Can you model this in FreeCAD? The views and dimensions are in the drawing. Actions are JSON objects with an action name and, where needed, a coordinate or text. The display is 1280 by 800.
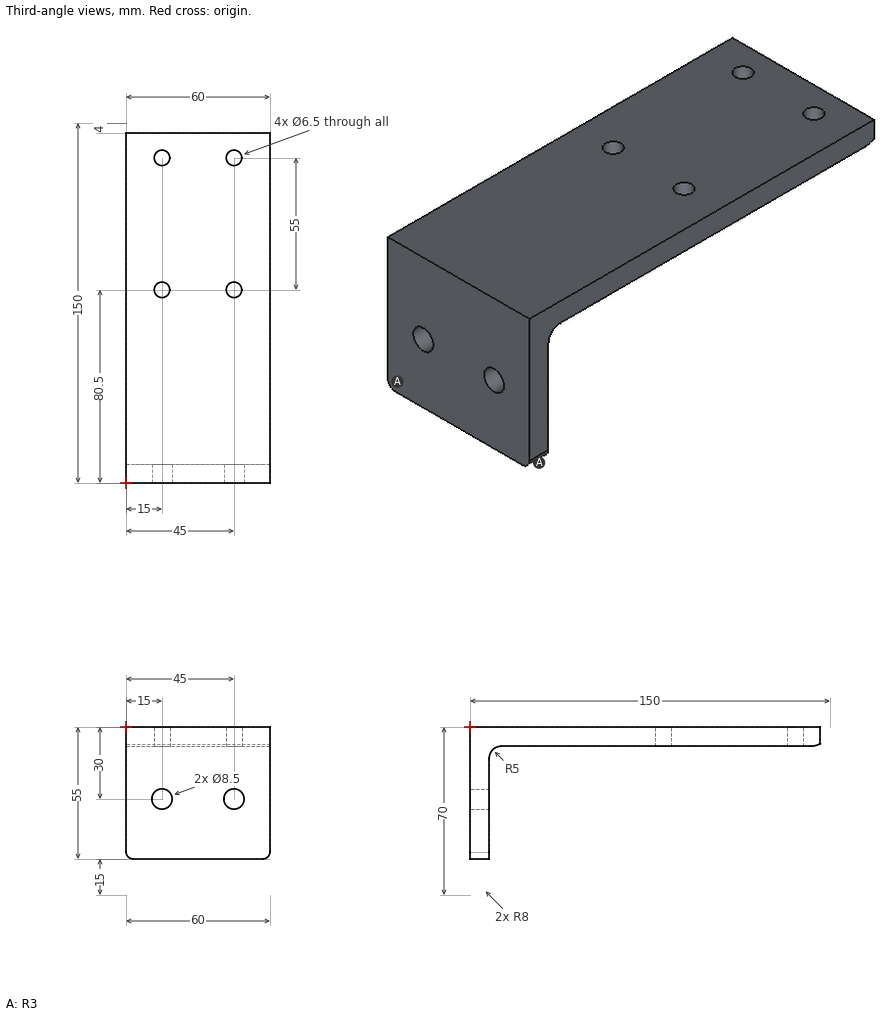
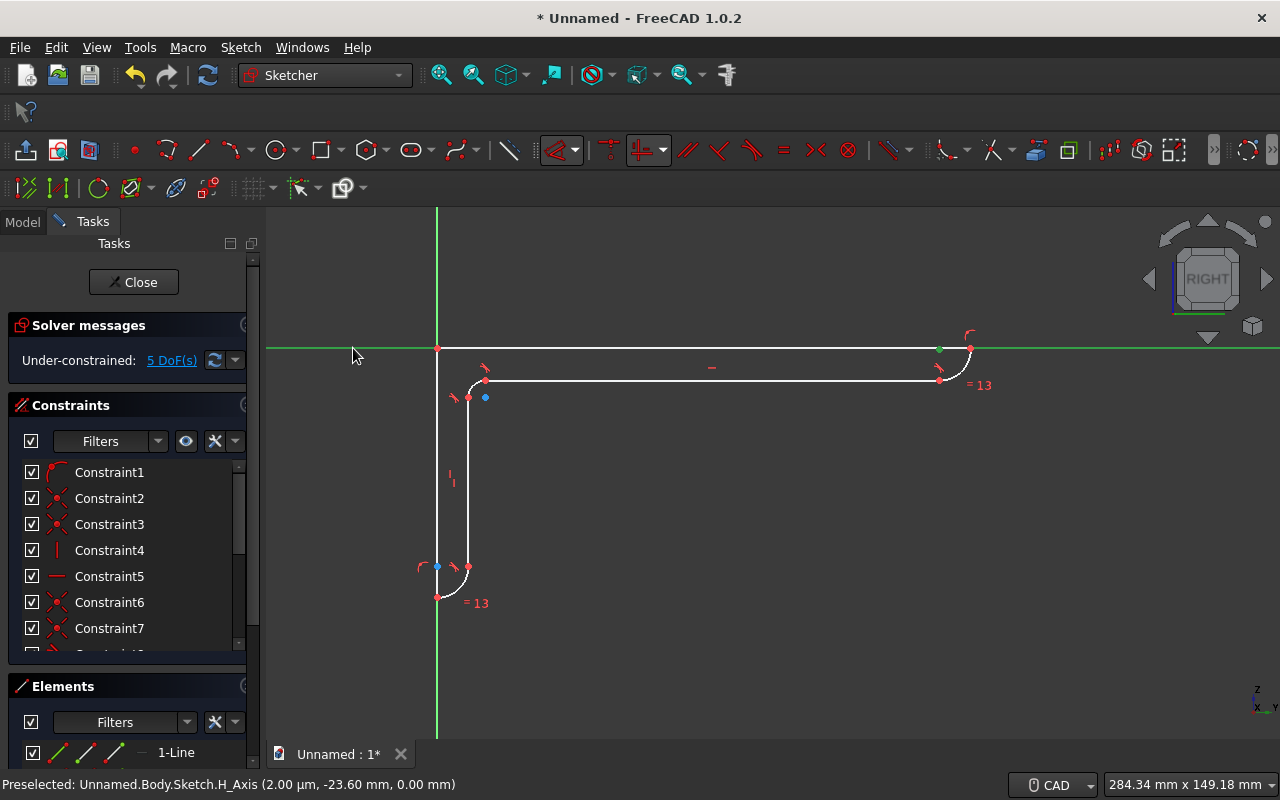
{"action": "key", "text": "c"}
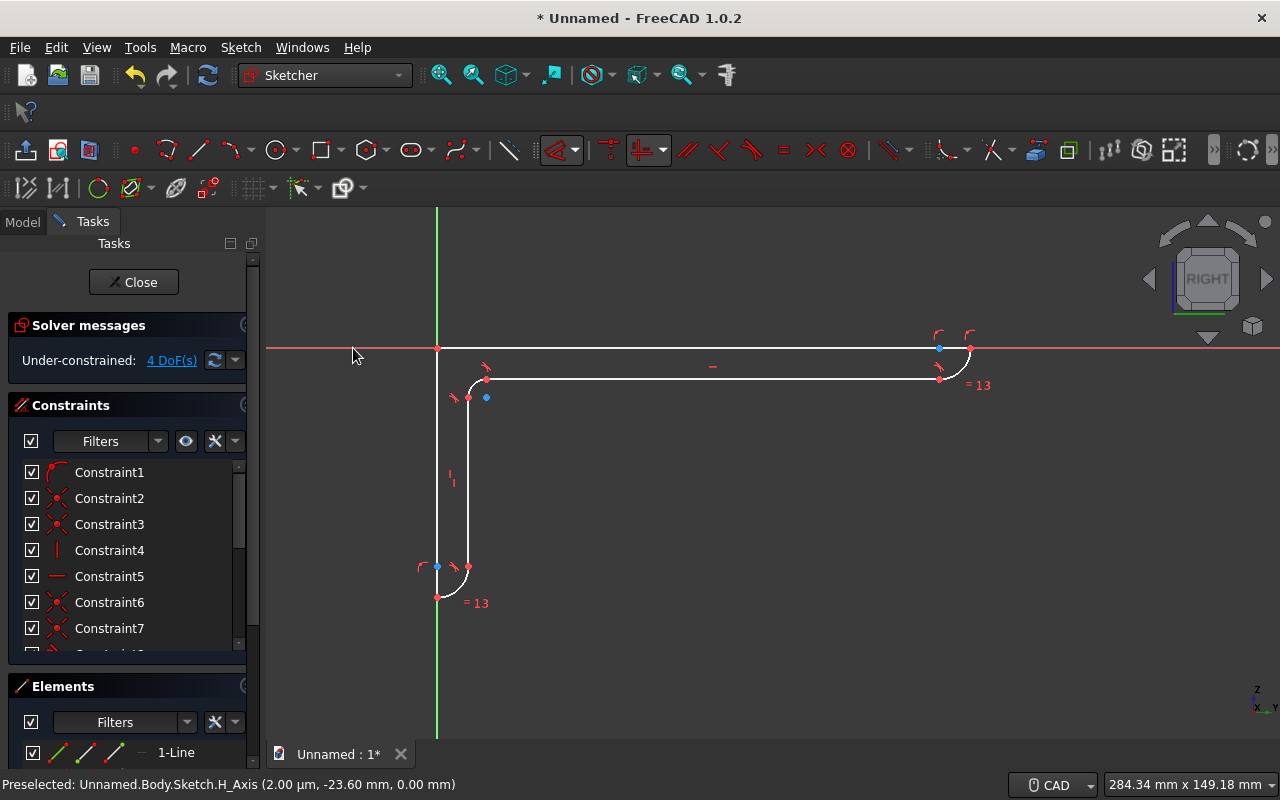
{"action": "key", "text": "d"}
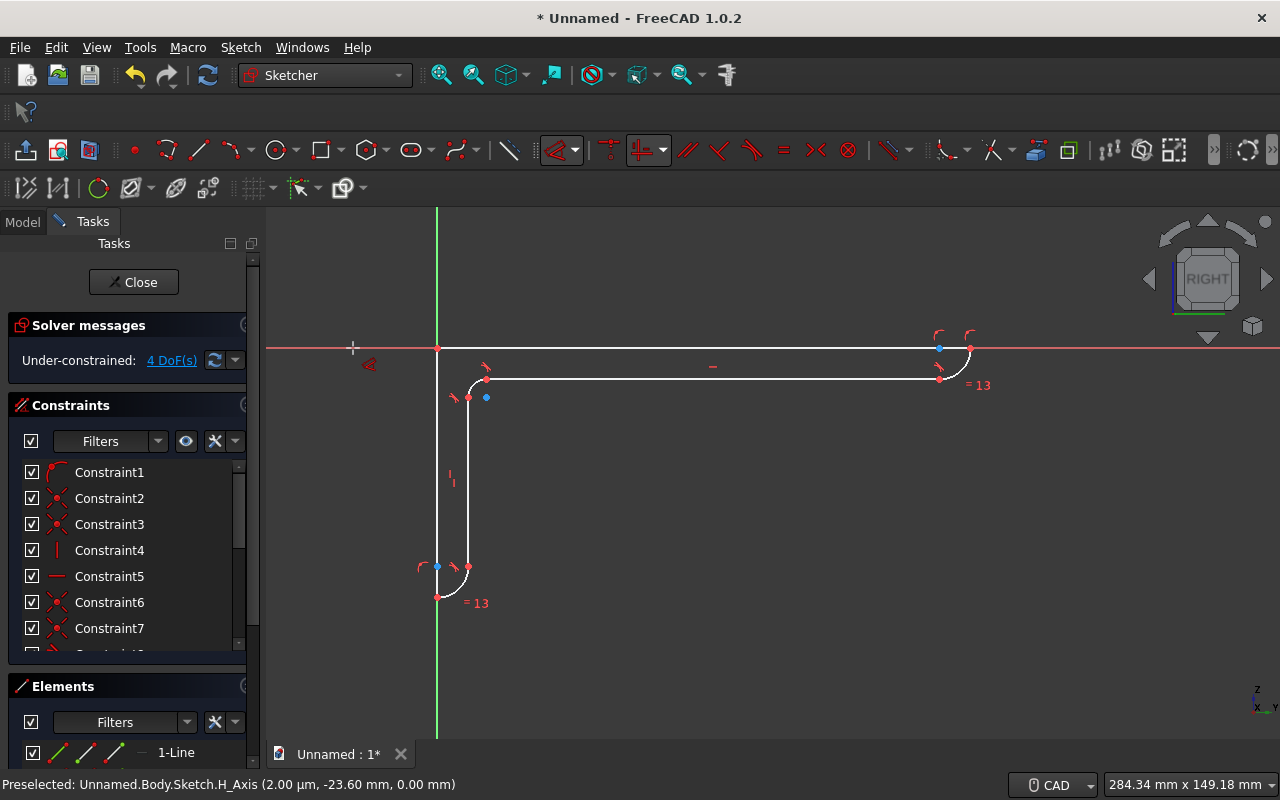
{"action": "scroll", "coordinate": [451, 594], "scroll_direction": "up", "scroll_amount": 2}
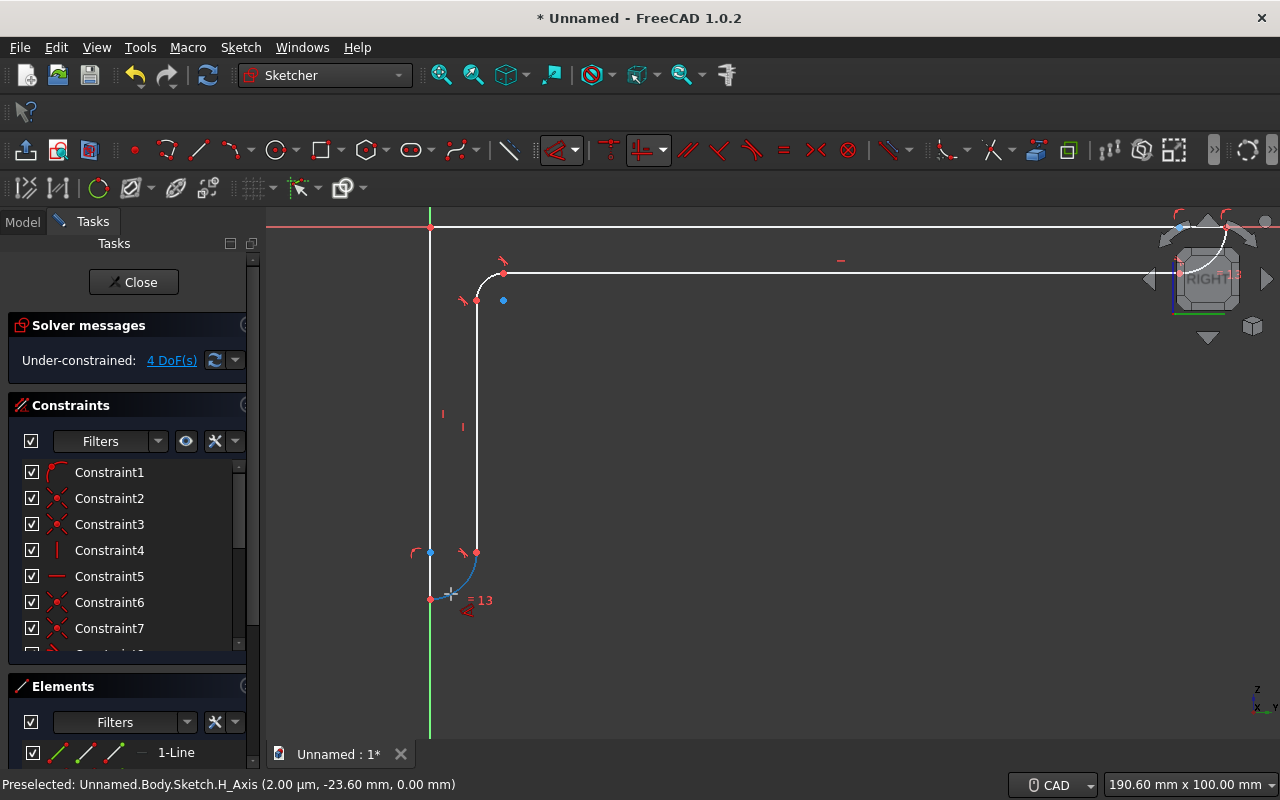
{"action": "left_click", "coordinate": [451, 594]}
{"action": "left_click", "coordinate": [465, 623]}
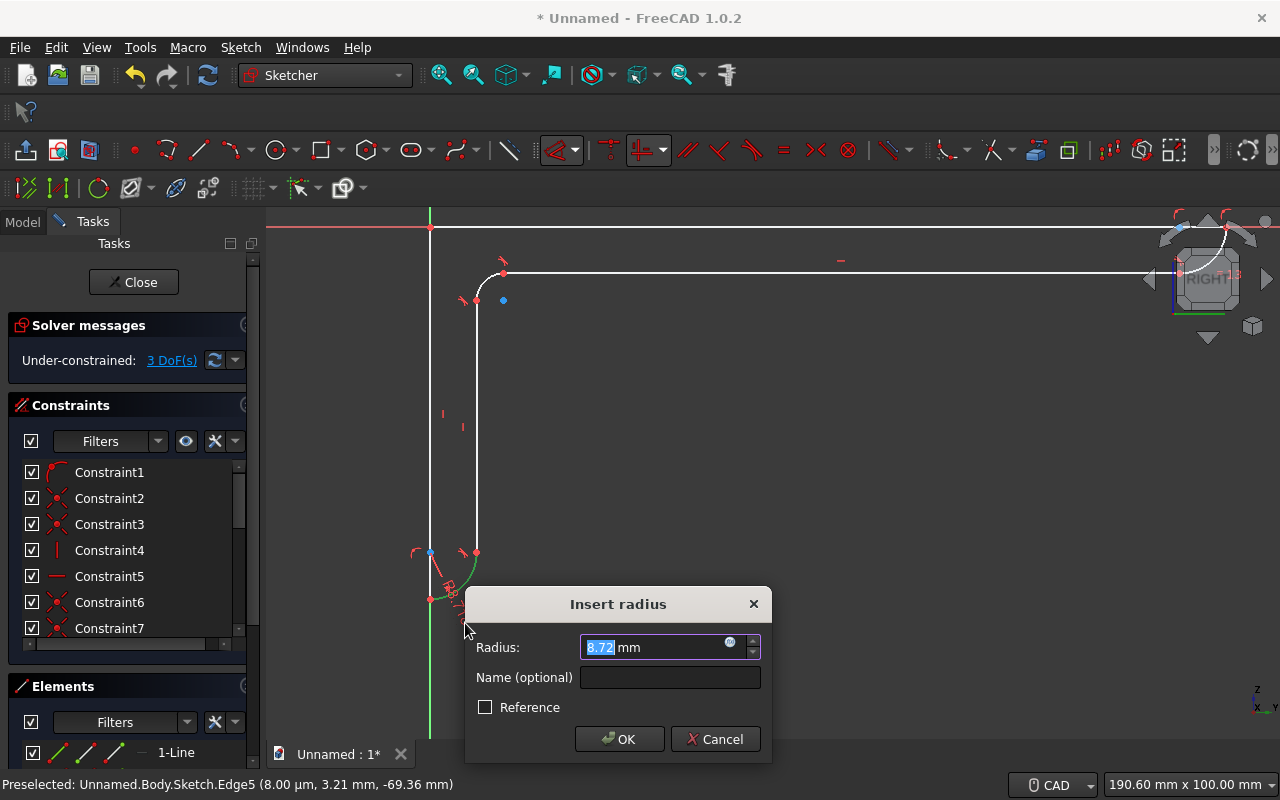
{"action": "type", "text": "8"}
{"action": "key", "text": "Return"}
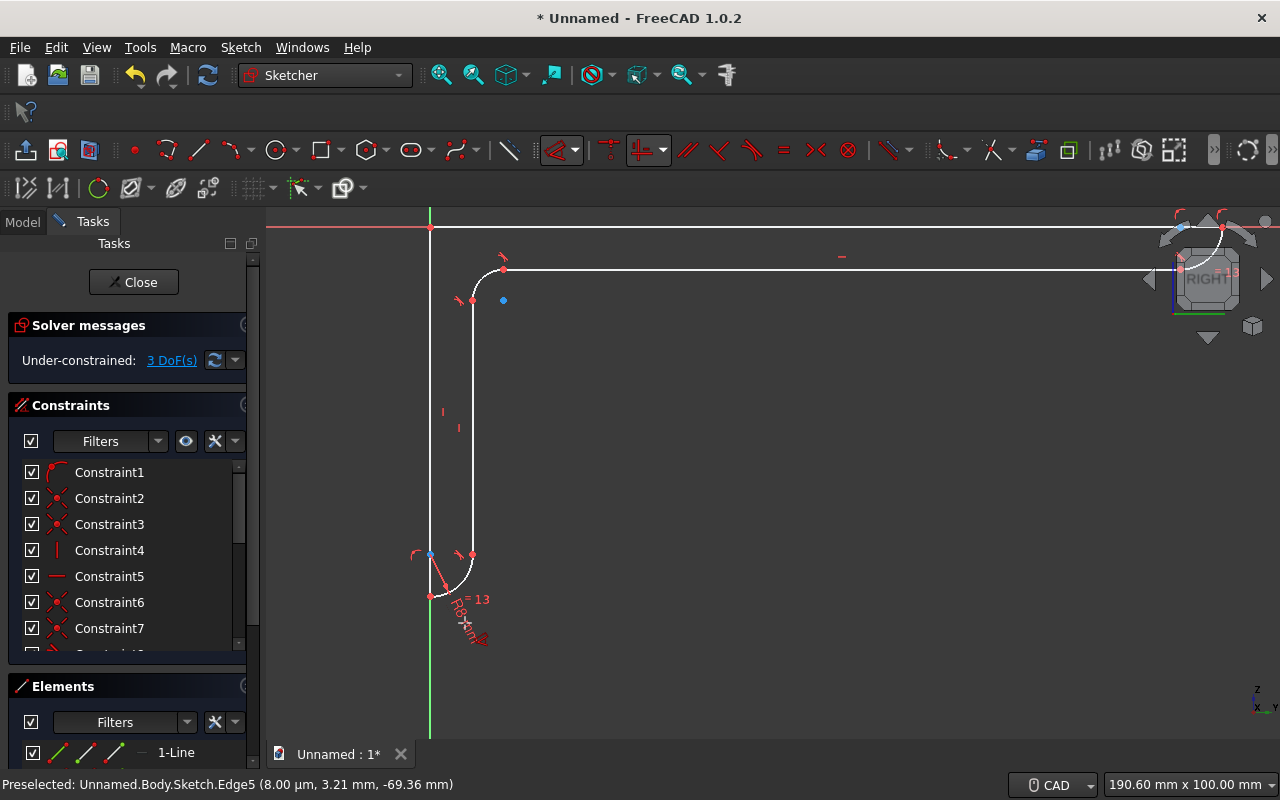
{"action": "scroll", "coordinate": [490, 273], "scroll_direction": "up", "scroll_amount": 3}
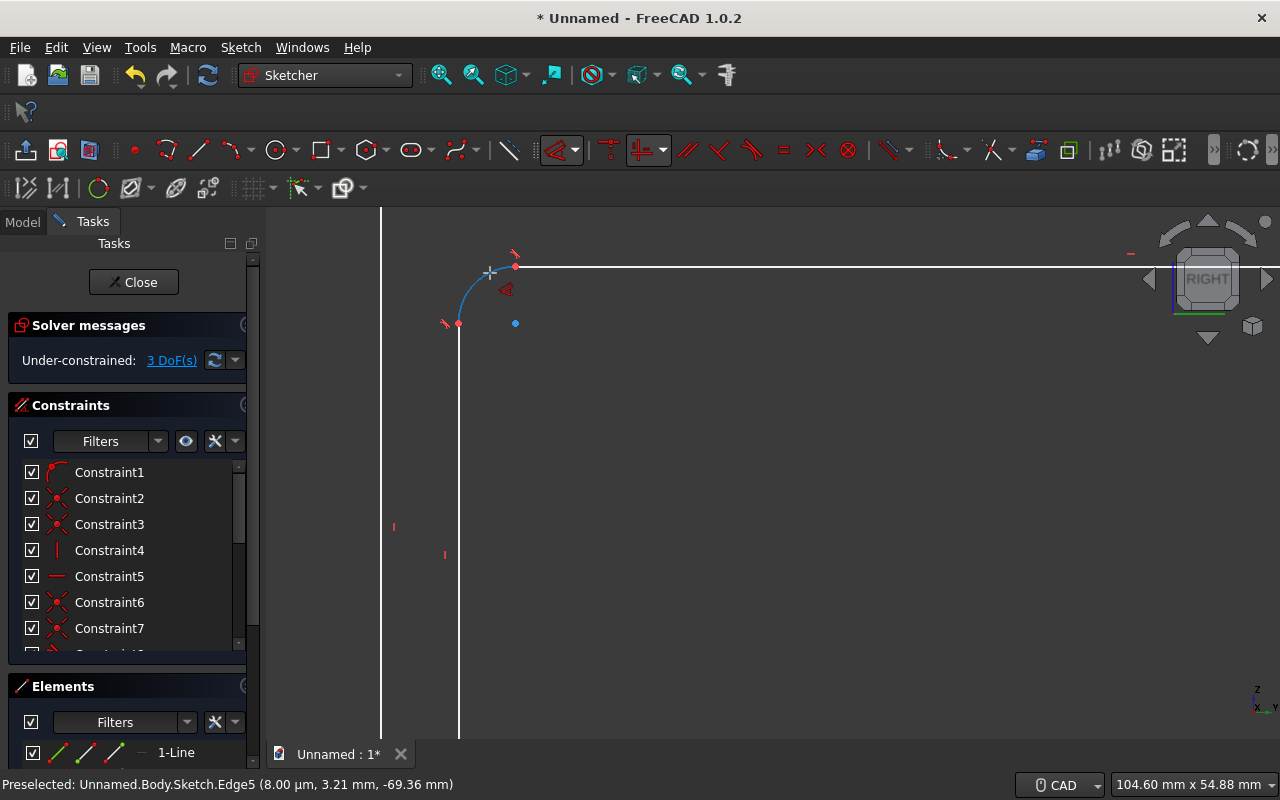
{"action": "left_click", "coordinate": [490, 273]}
{"action": "left_click", "coordinate": [476, 244]}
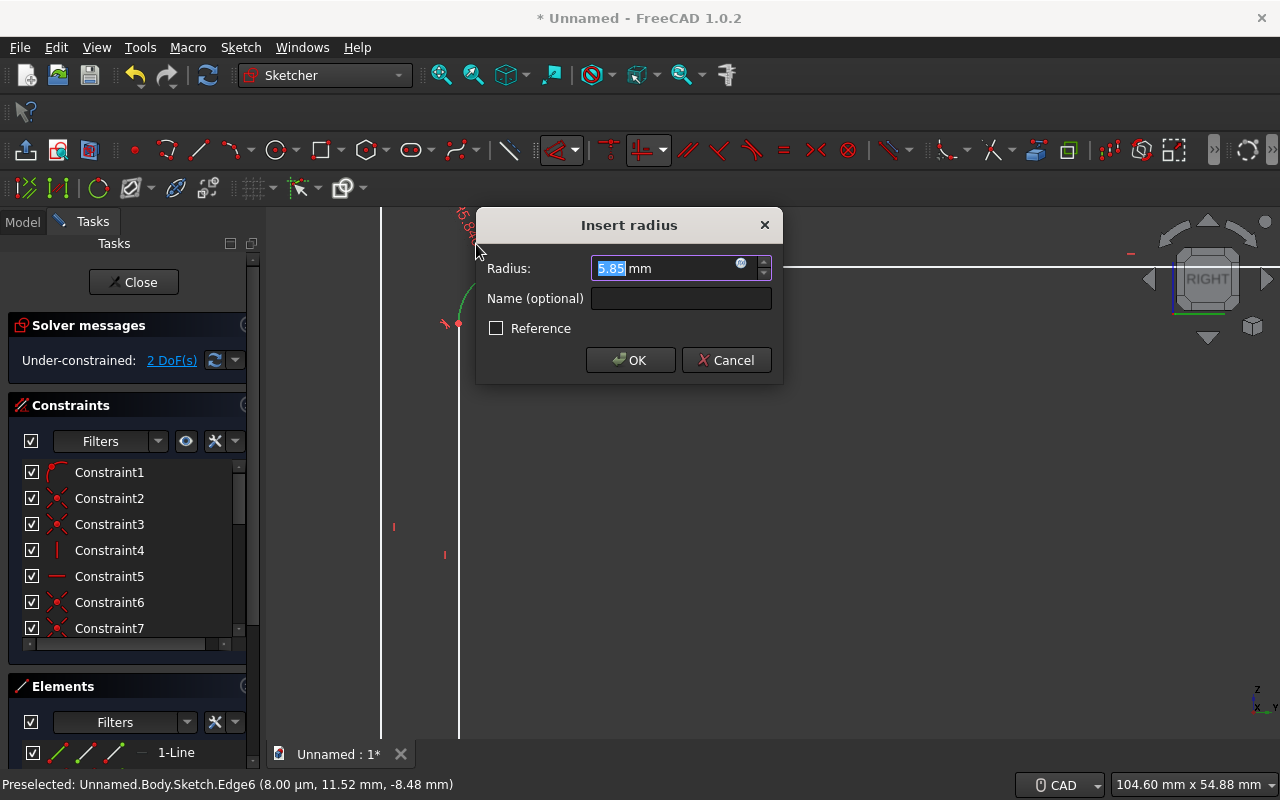
{"action": "type", "text": "5"}
{"action": "key", "text": "Return"}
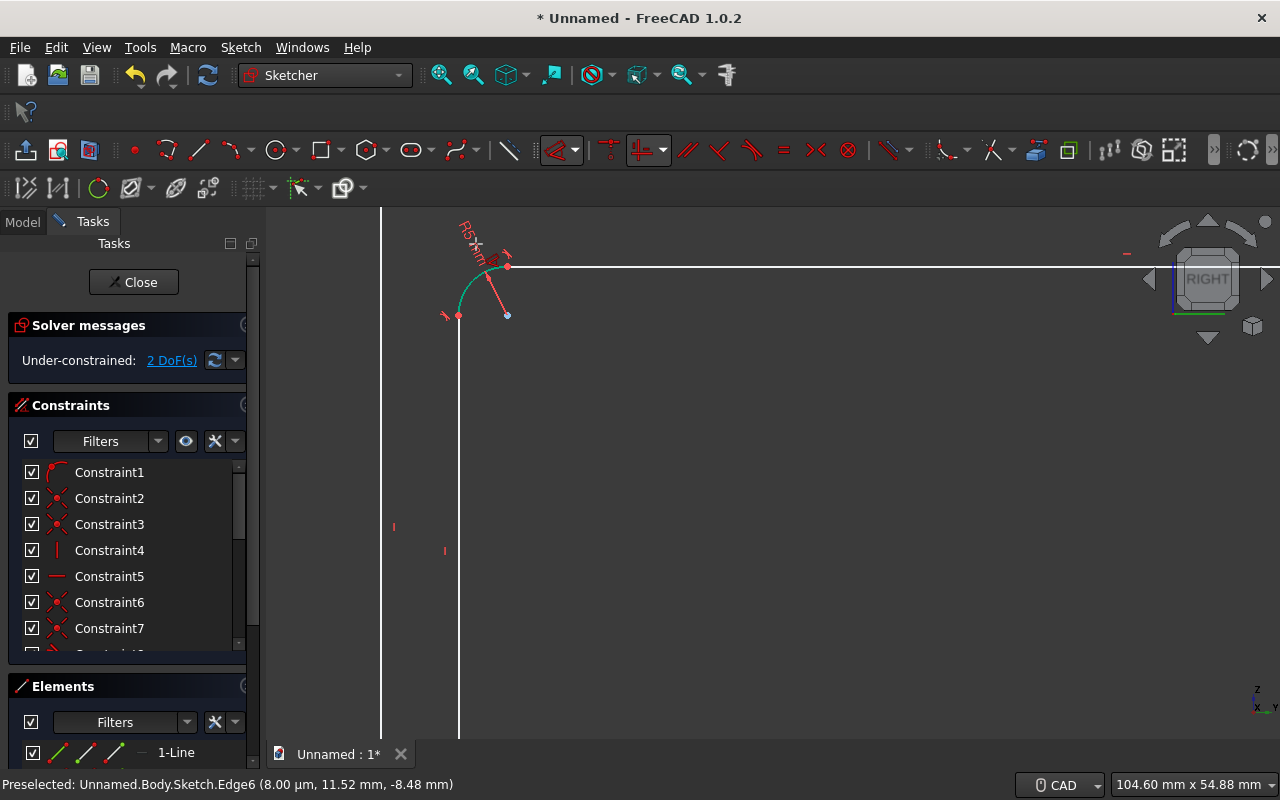
{"action": "left_click", "coordinate": [381, 391]}
{"action": "left_click", "coordinate": [347, 473]}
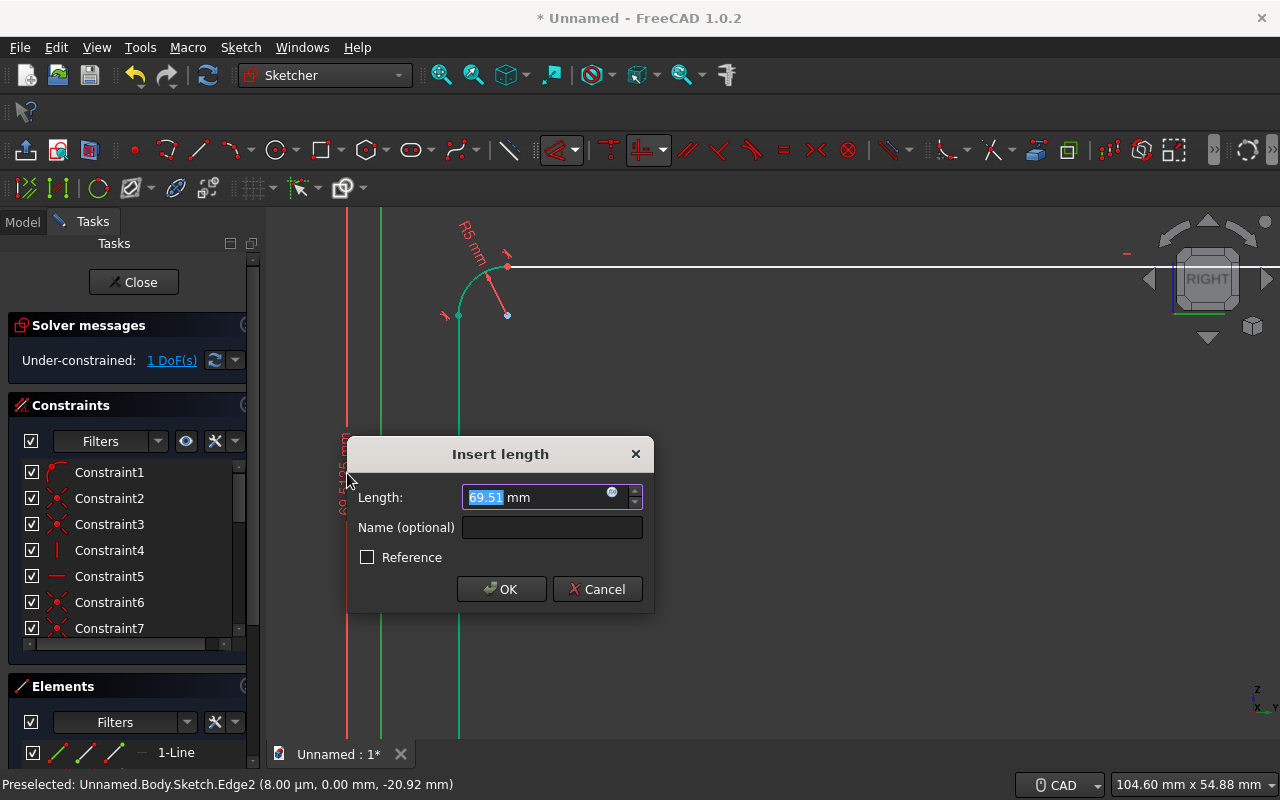
{"action": "type", "text": "70"}
{"action": "key", "text": "Return"}